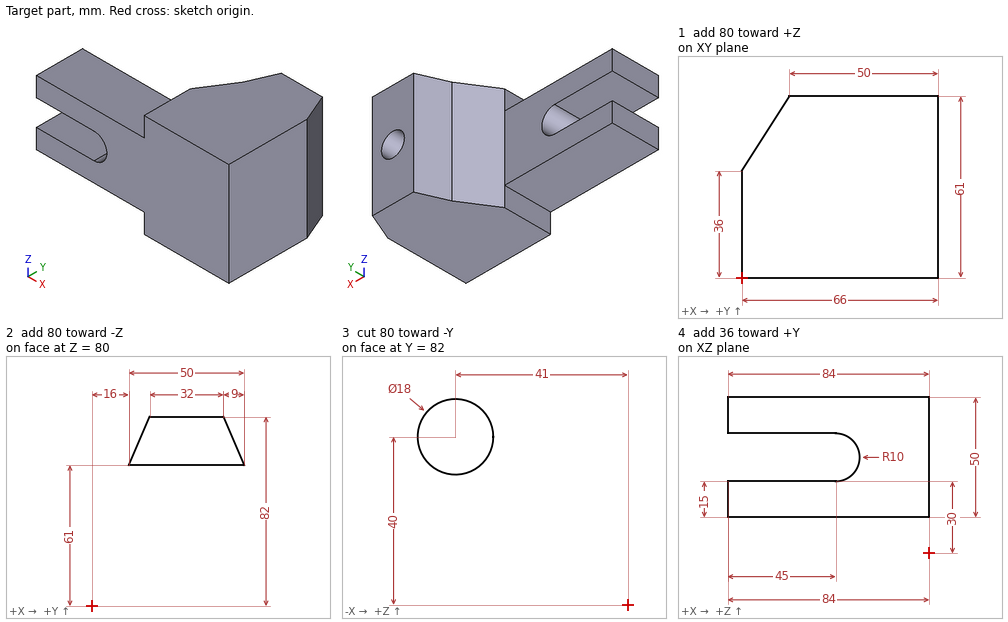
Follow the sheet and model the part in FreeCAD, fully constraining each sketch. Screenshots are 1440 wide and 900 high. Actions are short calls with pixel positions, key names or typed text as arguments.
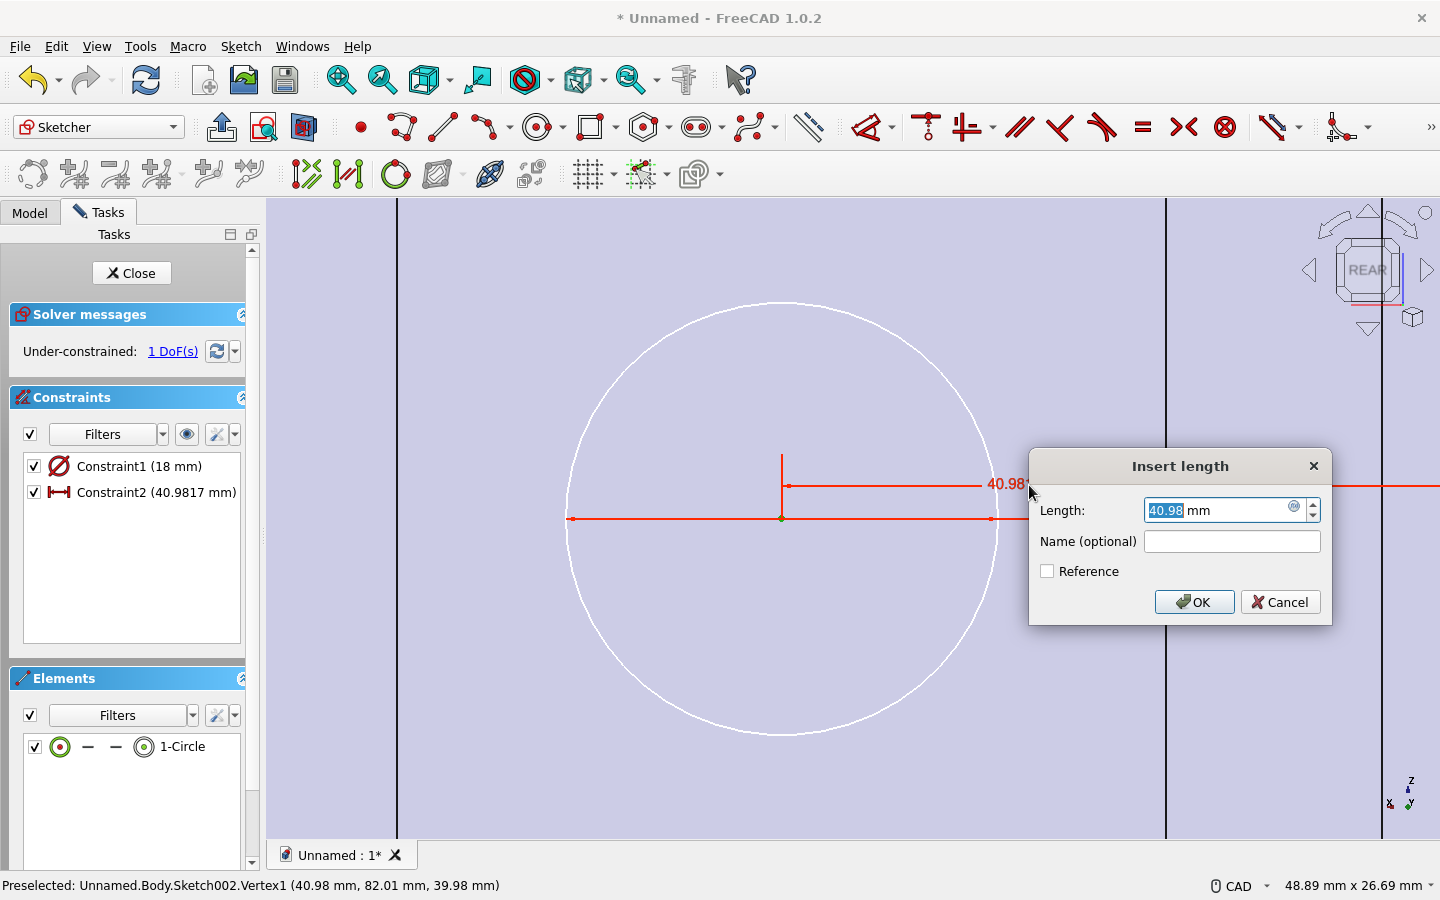
text(41)
key(Return)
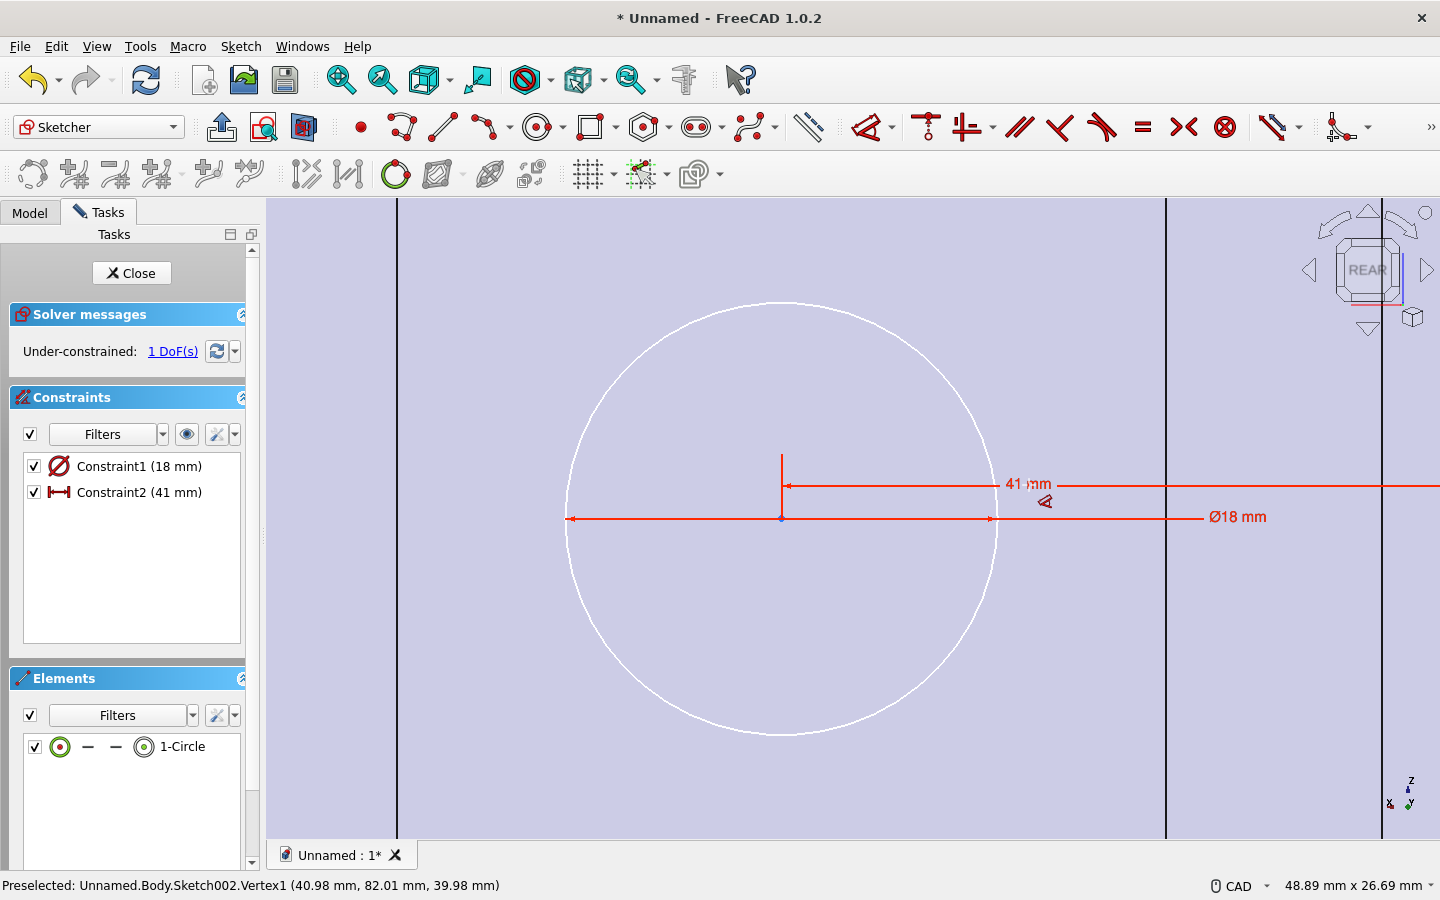
click(782, 519)
click(748, 665)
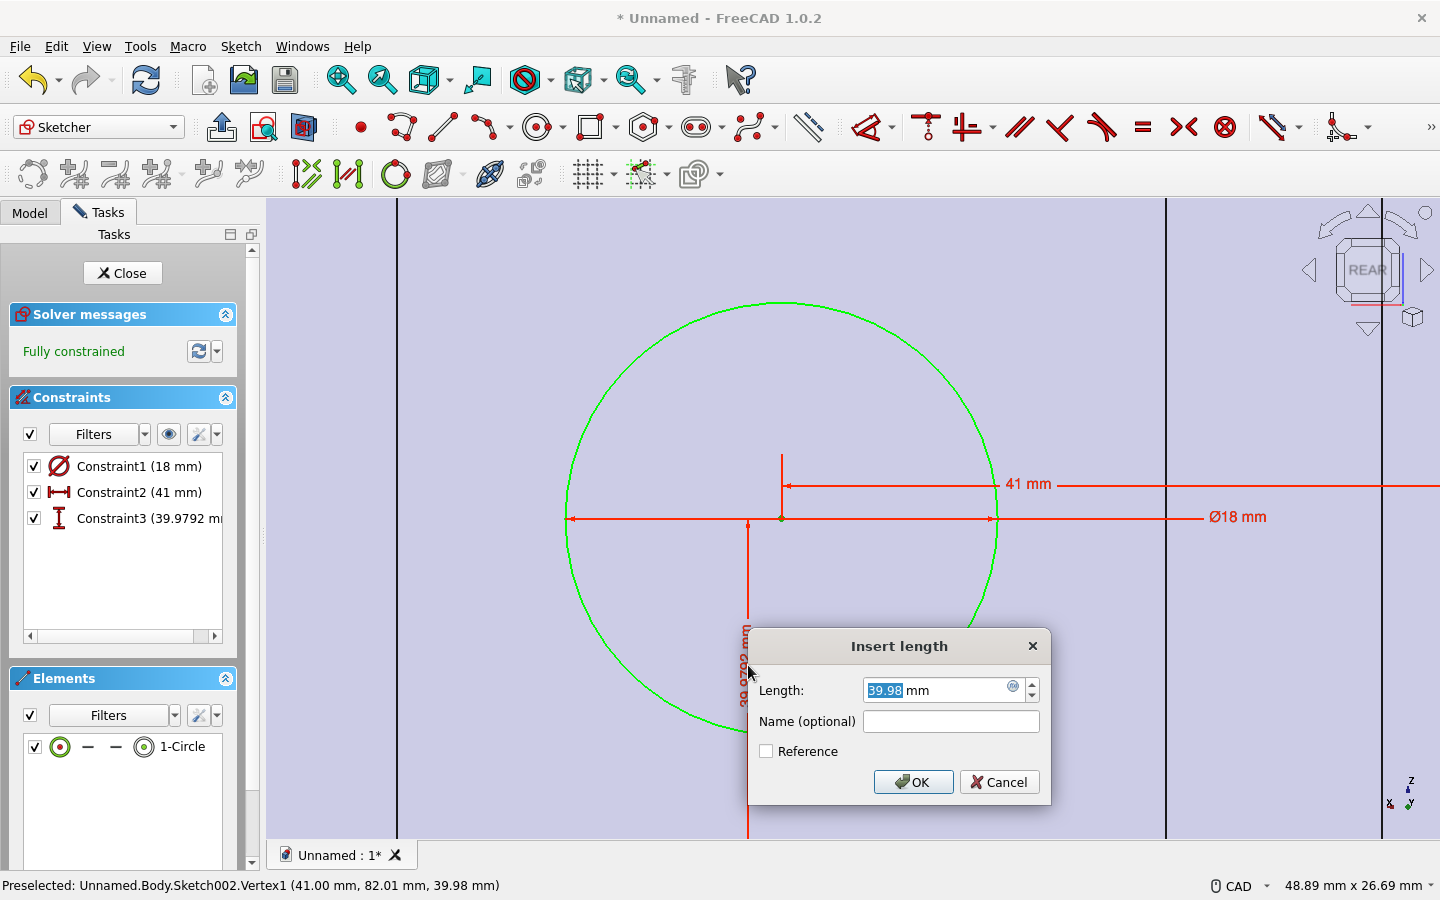
text(40)
key(Return)
key(Escape)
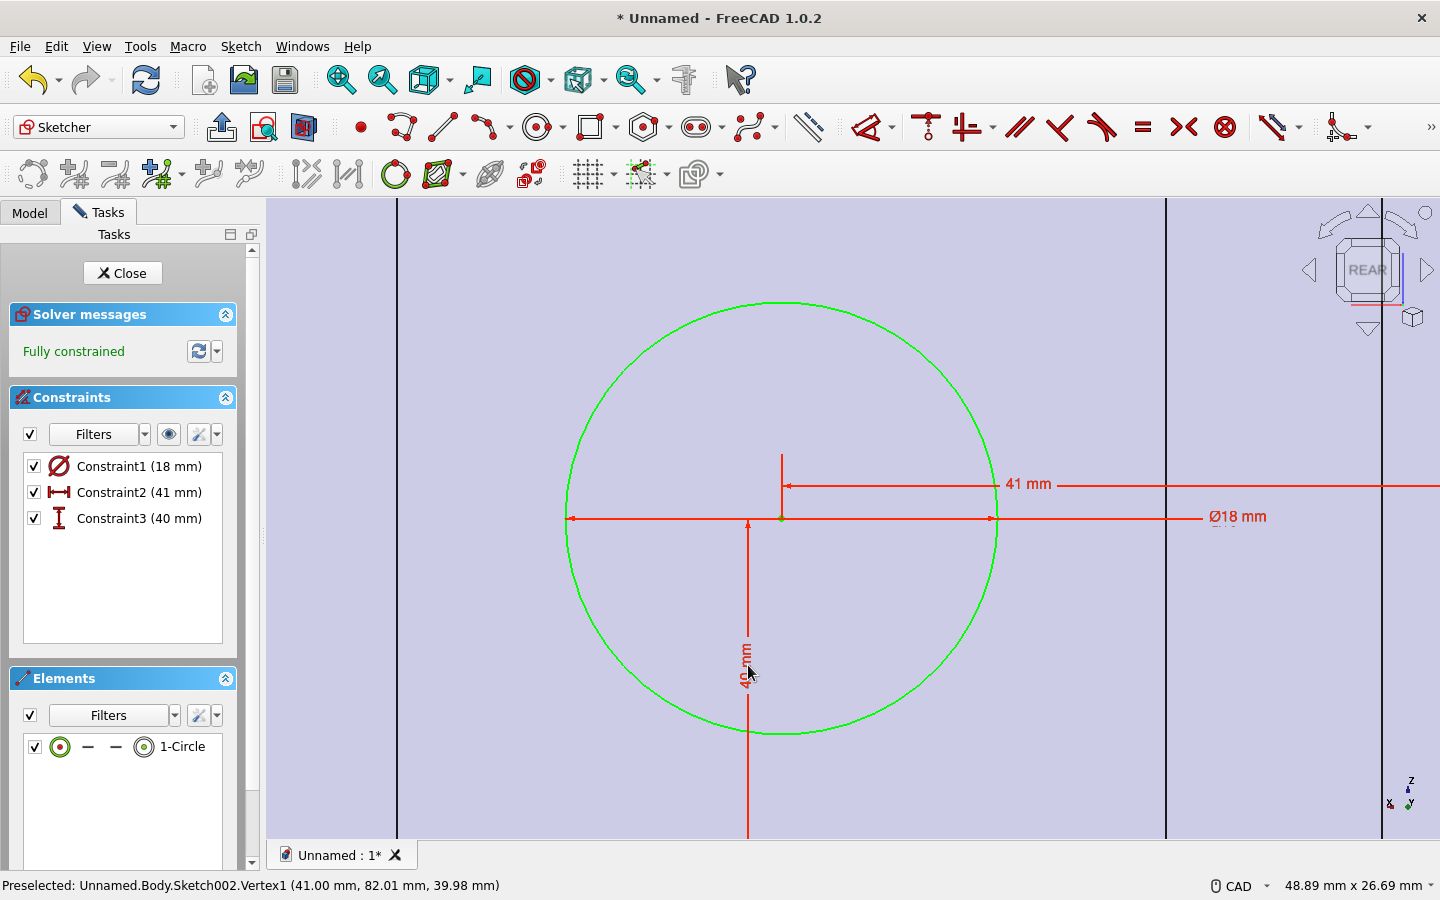
click(123, 273)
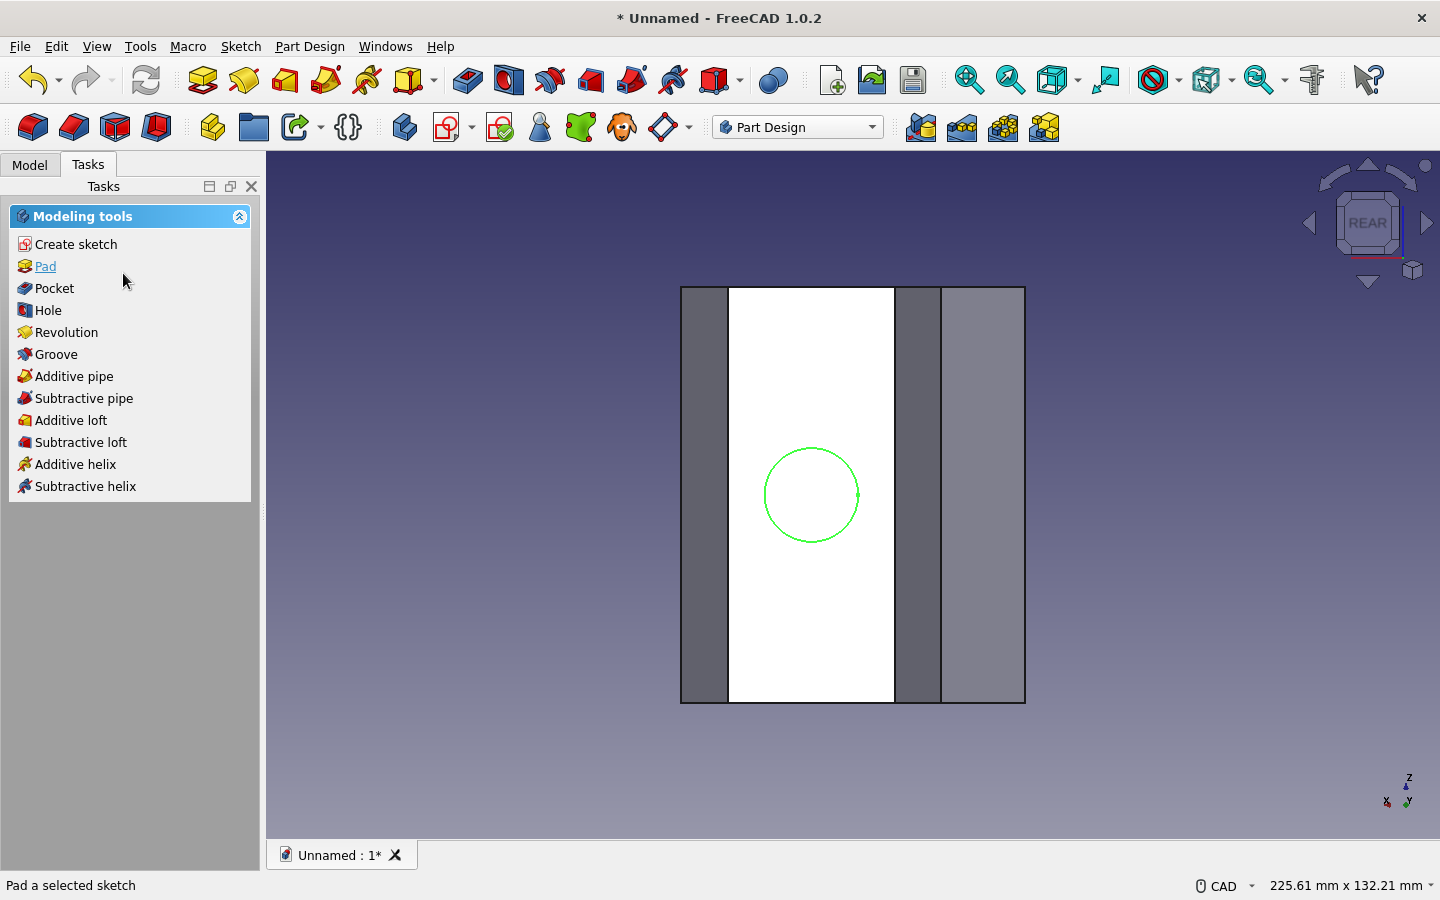
click(468, 80)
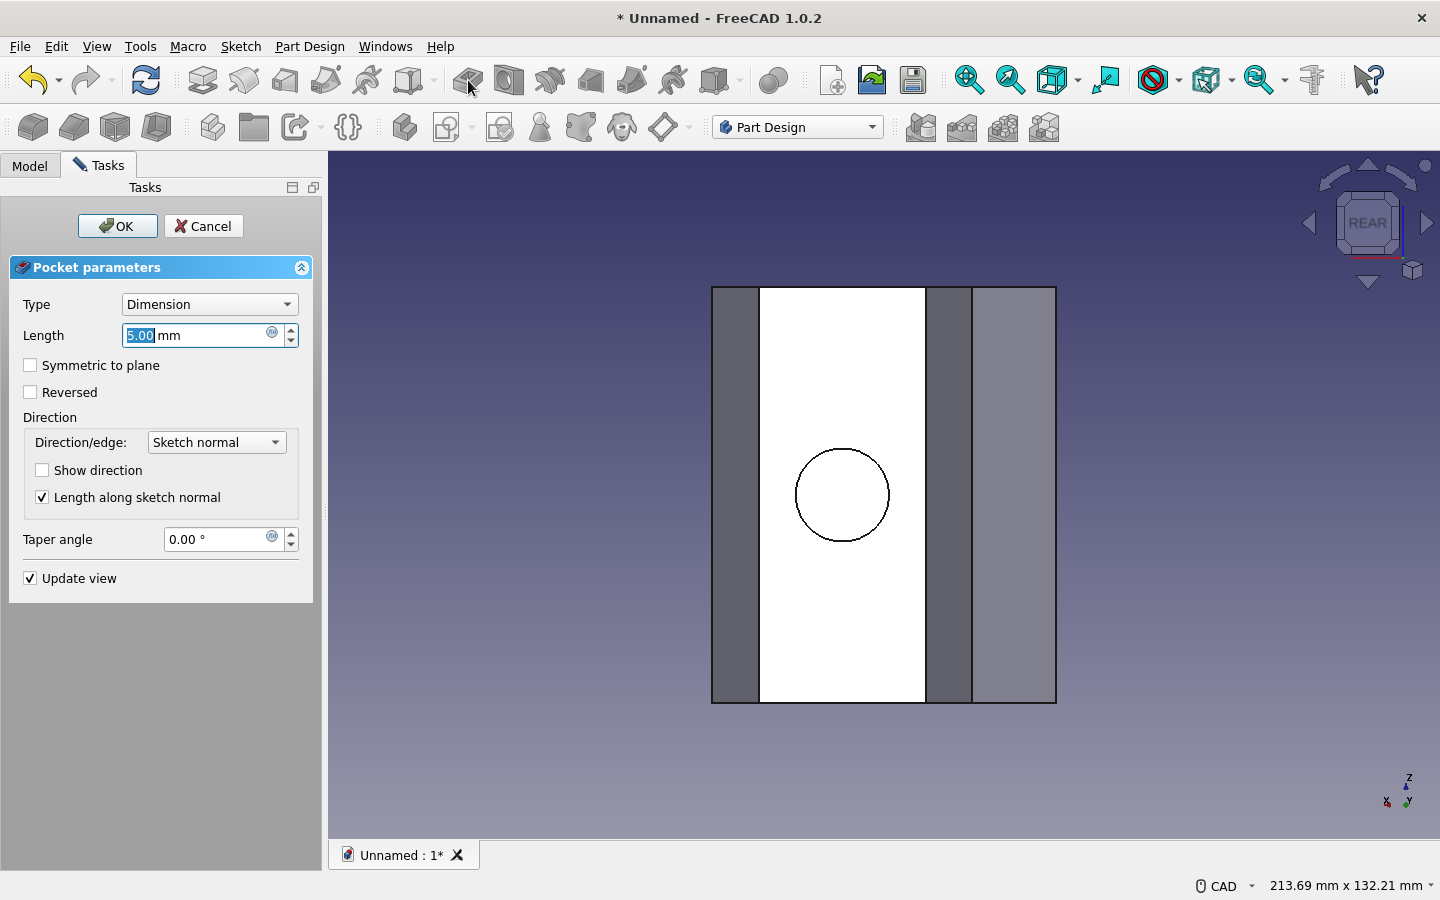
text(80)
key(Tab)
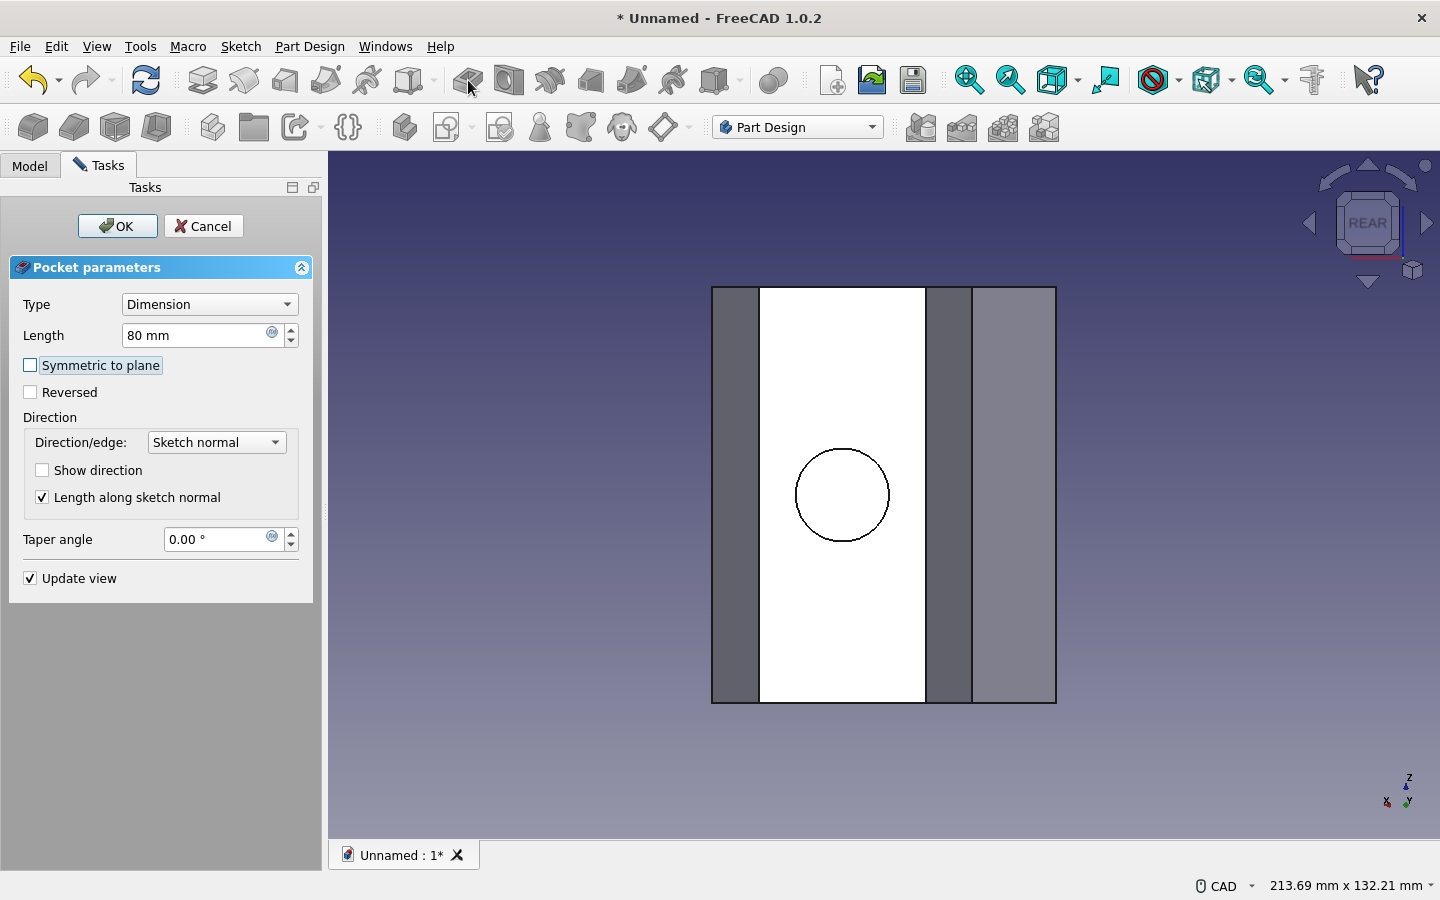
click(118, 226)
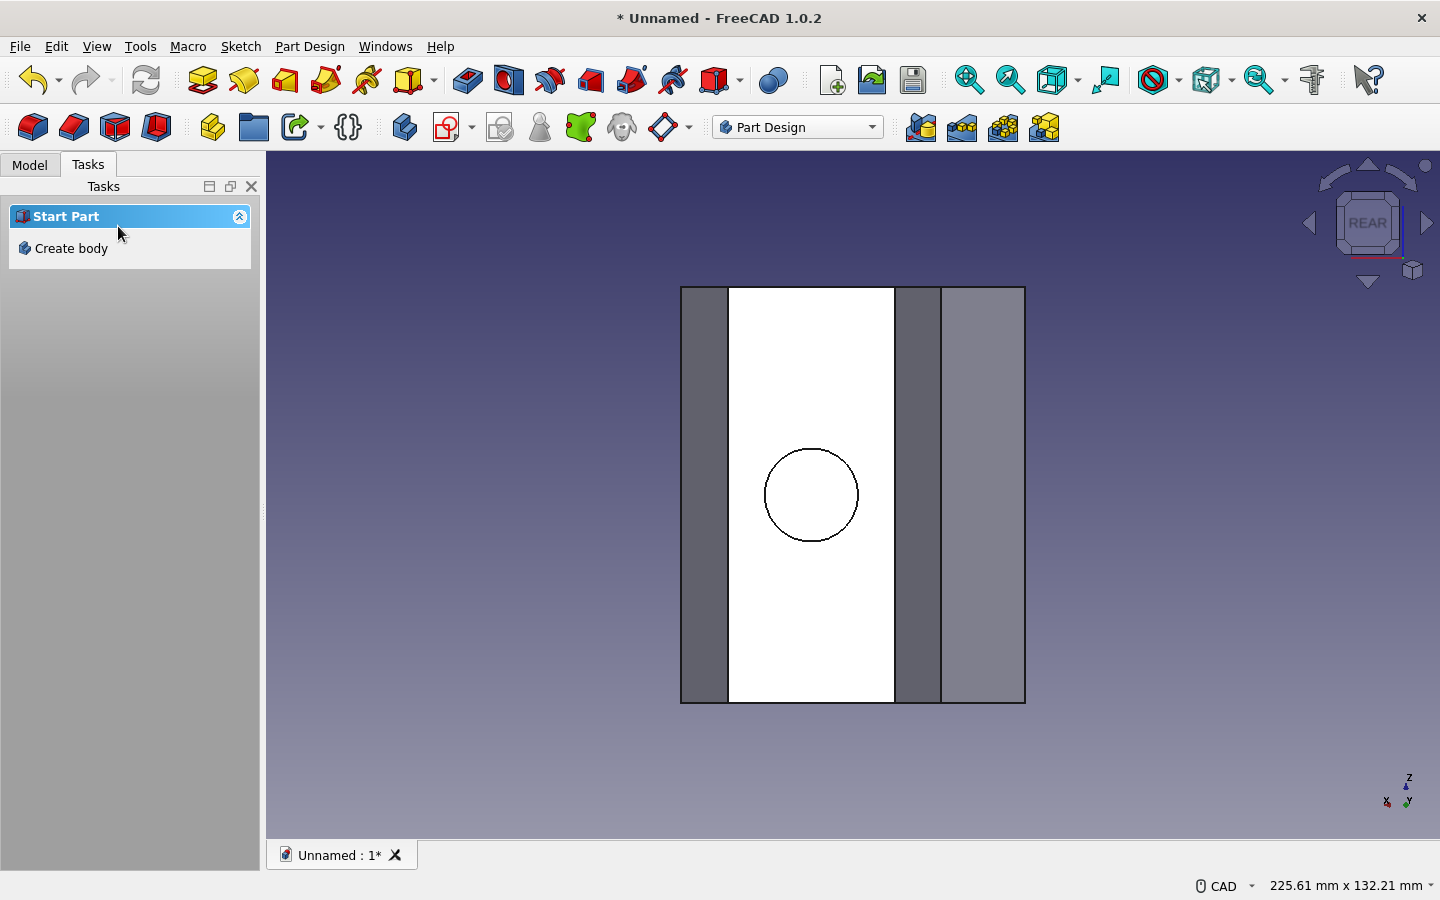
click(446, 128)